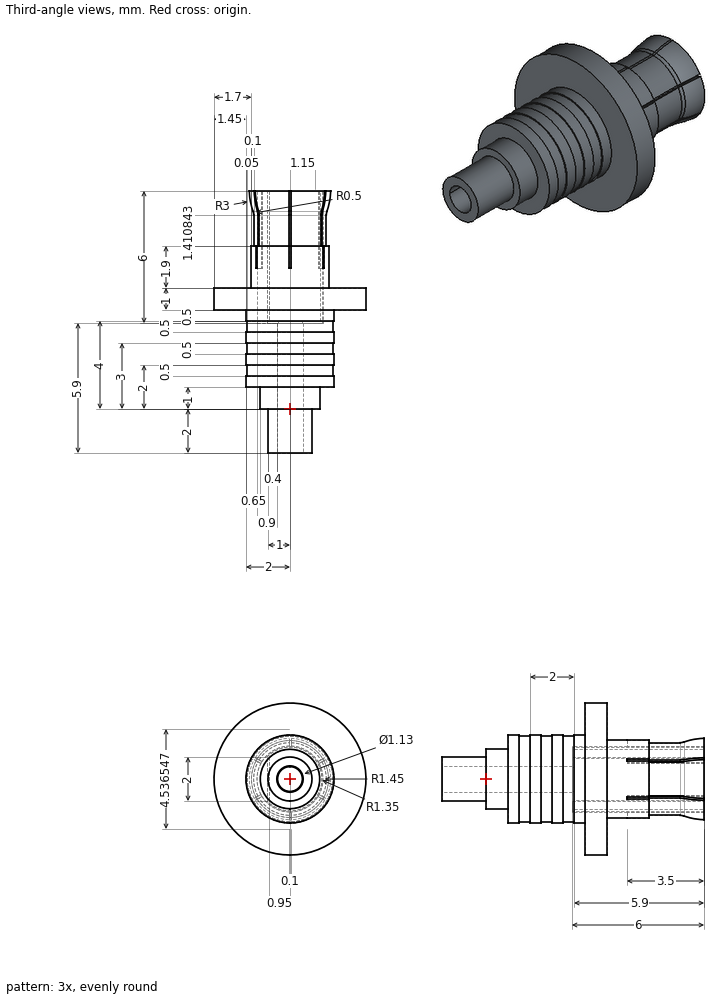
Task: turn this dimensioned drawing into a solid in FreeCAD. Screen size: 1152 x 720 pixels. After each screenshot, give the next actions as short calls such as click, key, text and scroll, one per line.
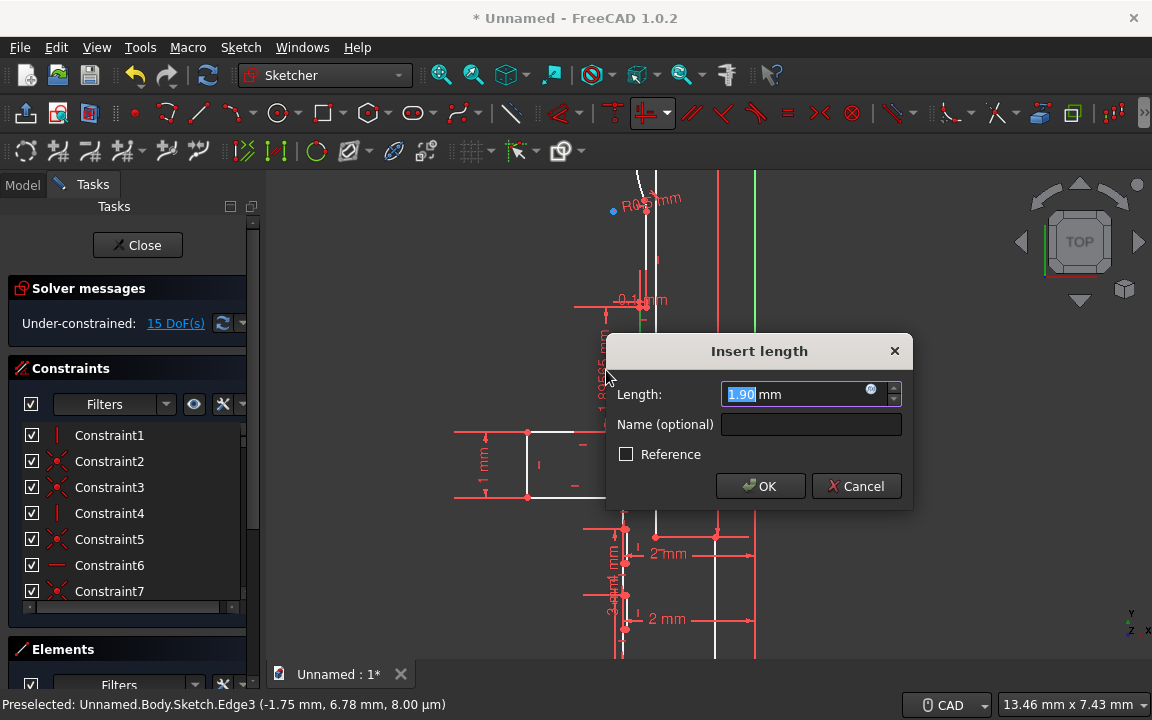
text(1.9)
key(Return)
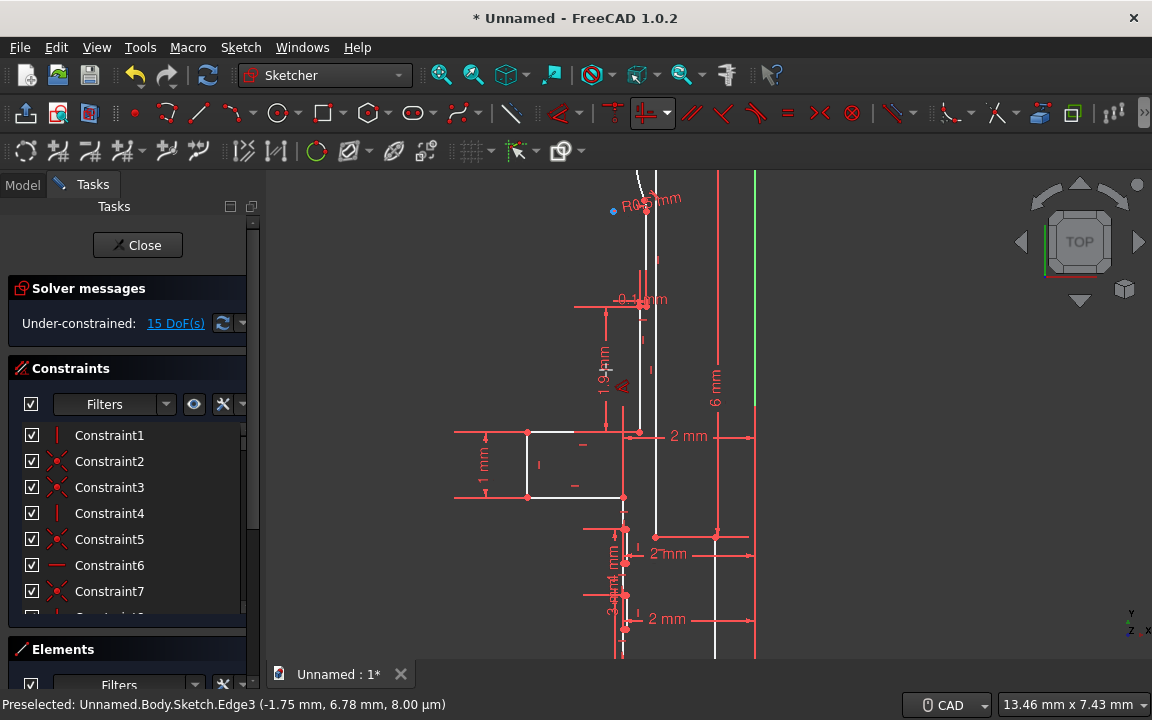
click(606, 432)
click(583, 398)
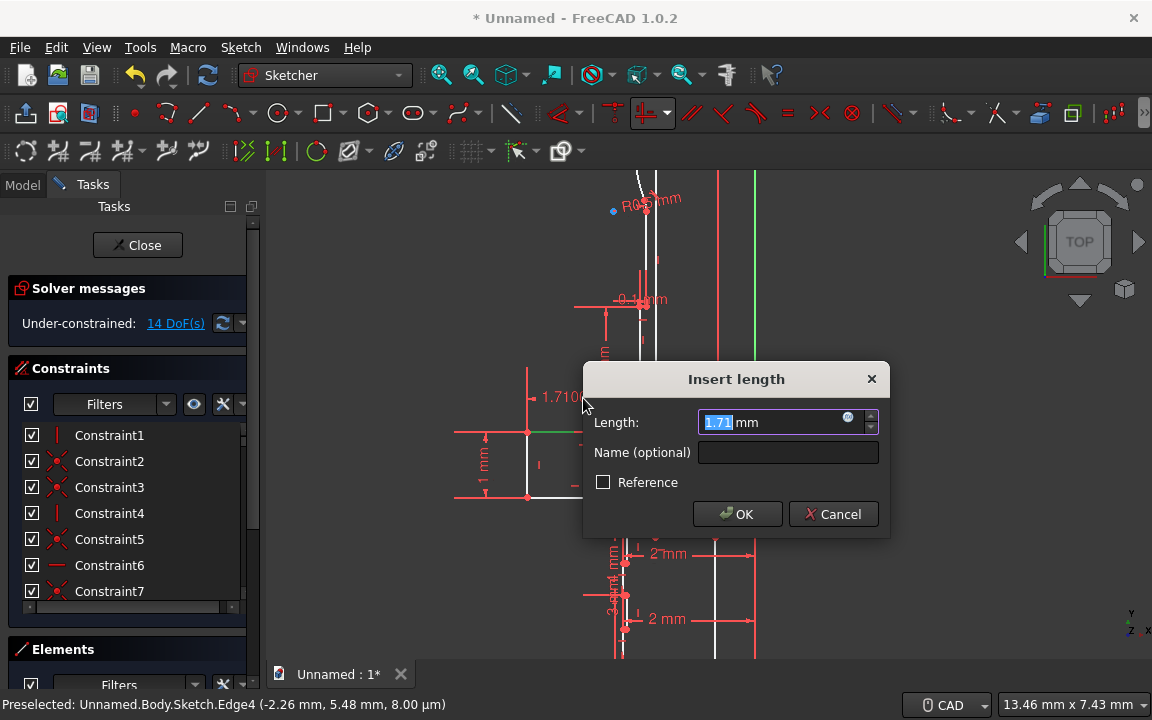
text(1.7)
key(Return)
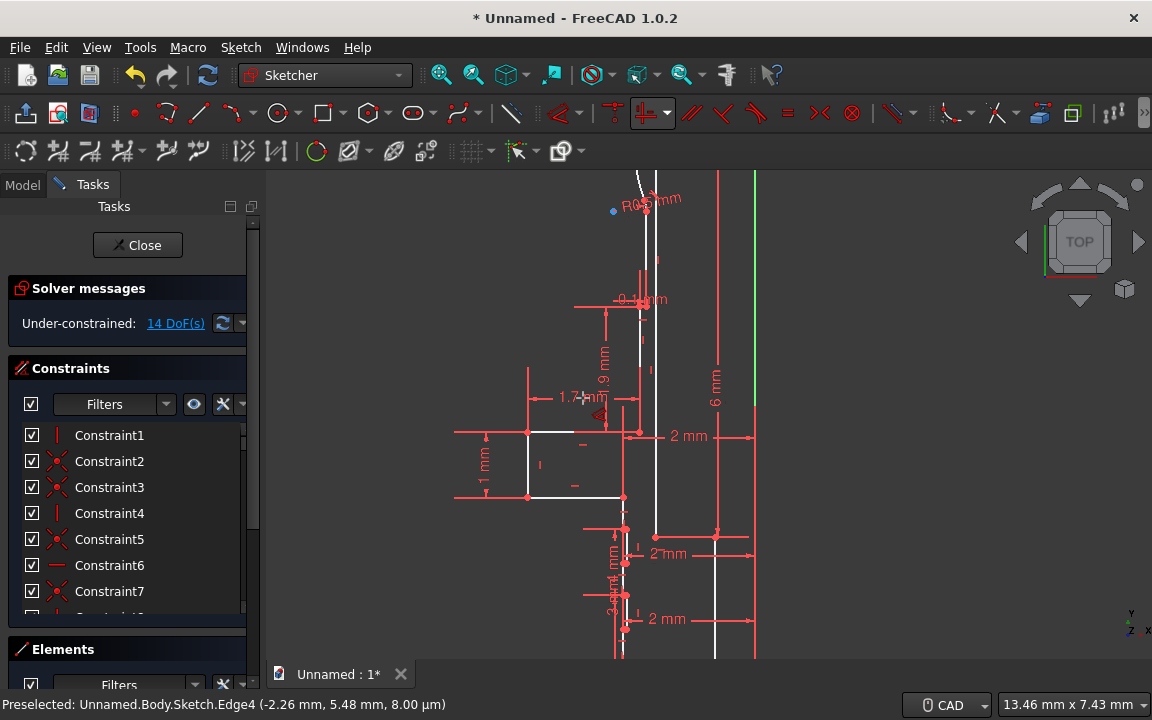
scroll(623, 507, up, 2)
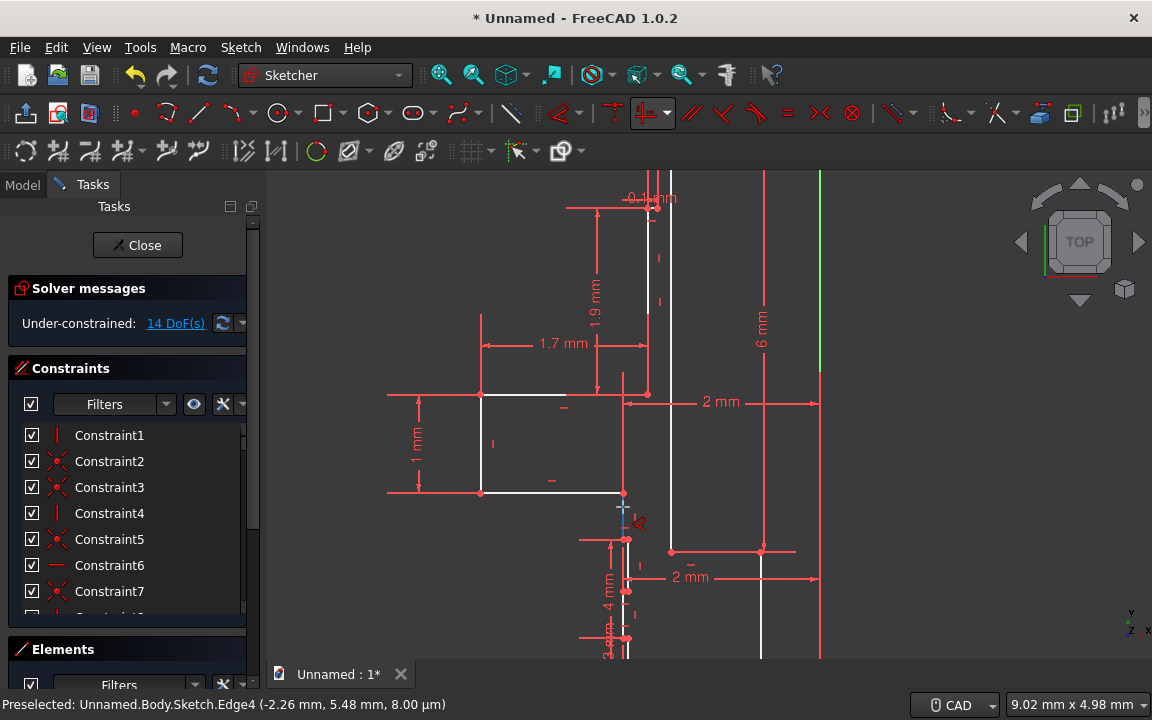
click(623, 507)
click(589, 516)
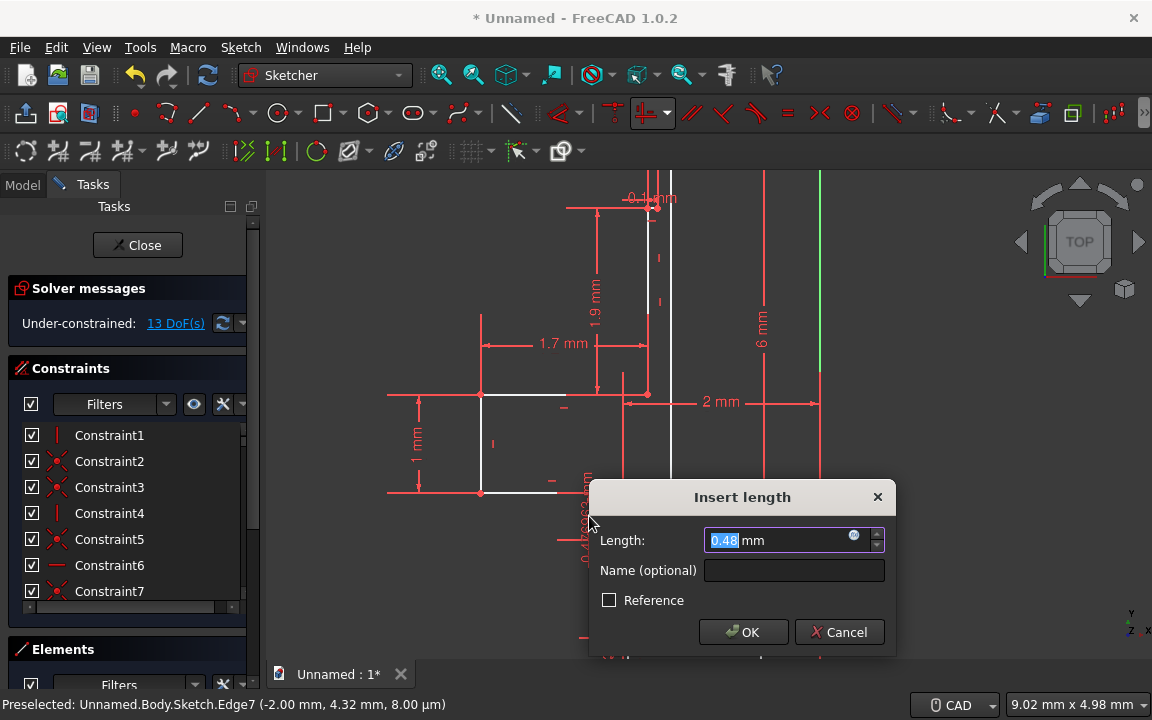
text(0.5)
key(Return)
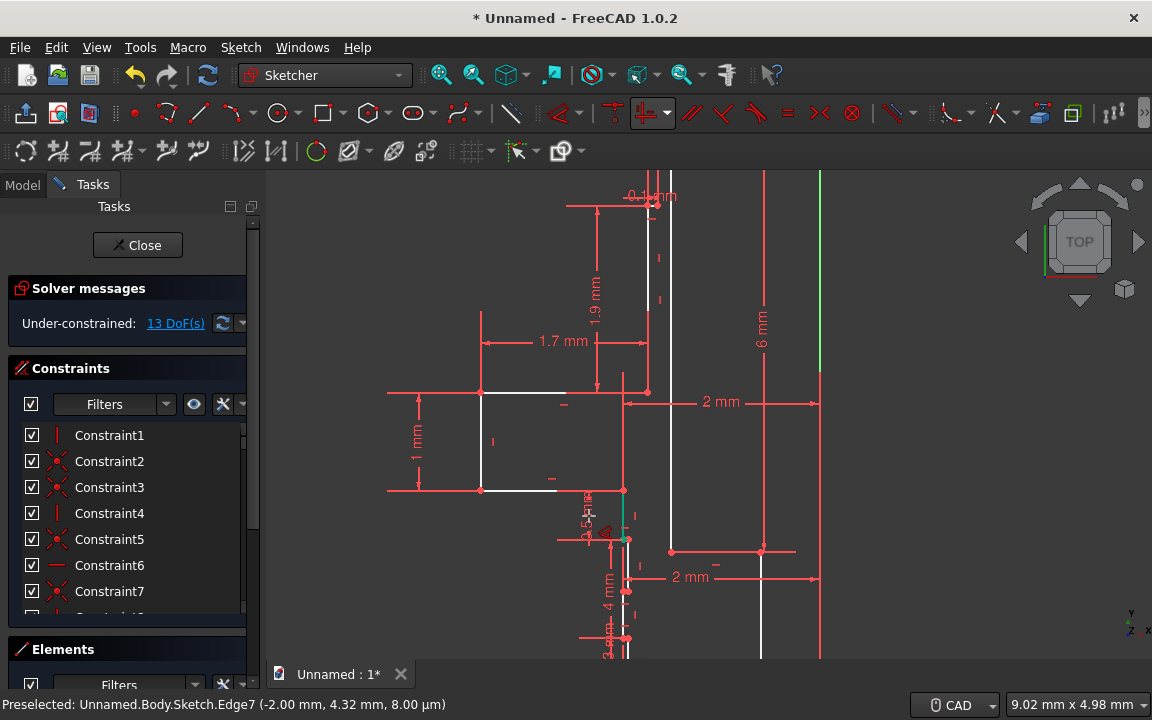
click(628, 555)
click(594, 566)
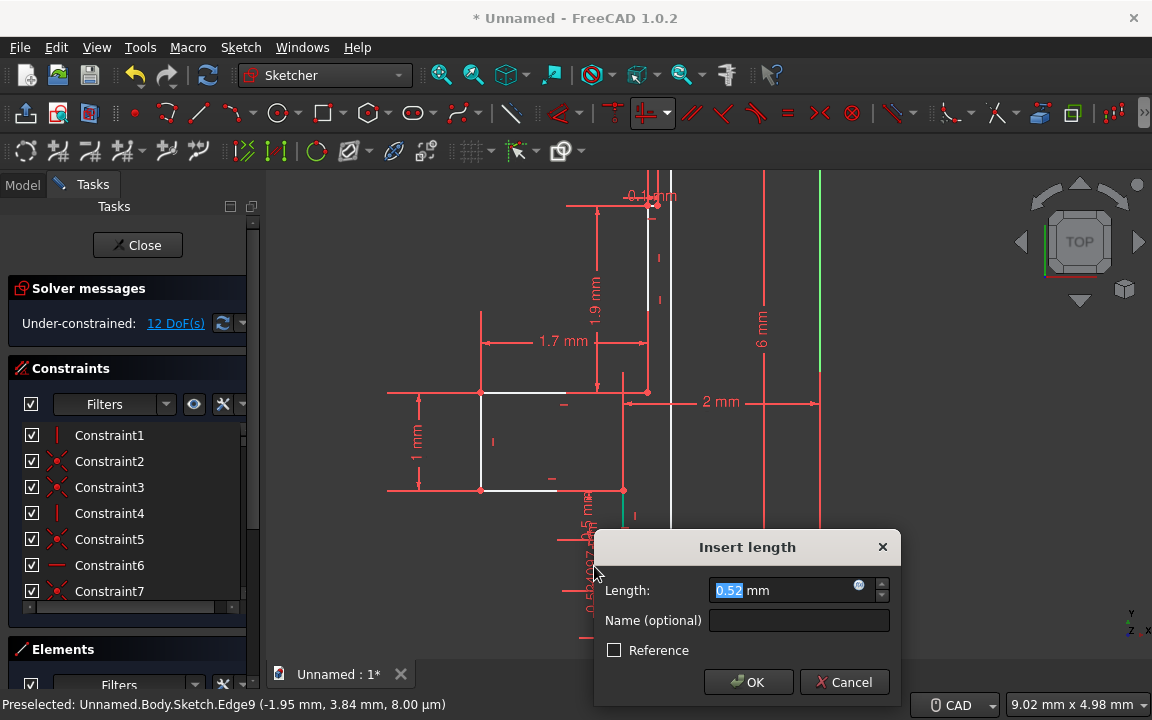
text(0.5)
key(Return)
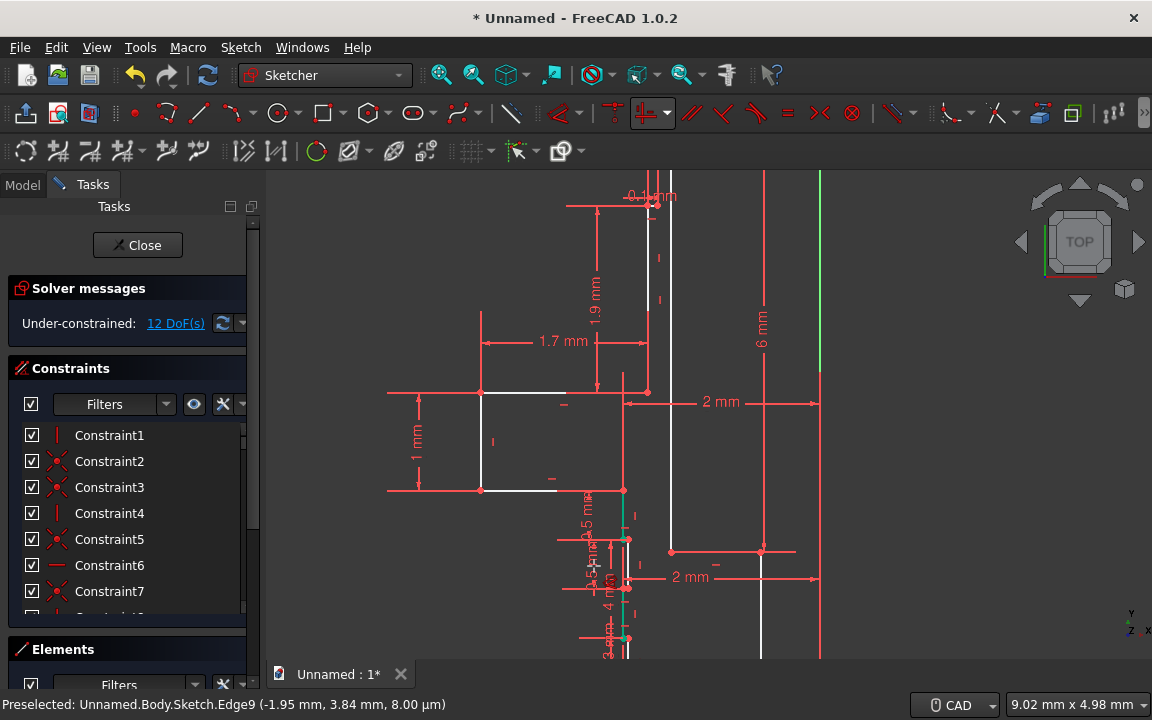
scroll(637, 372, down, 7)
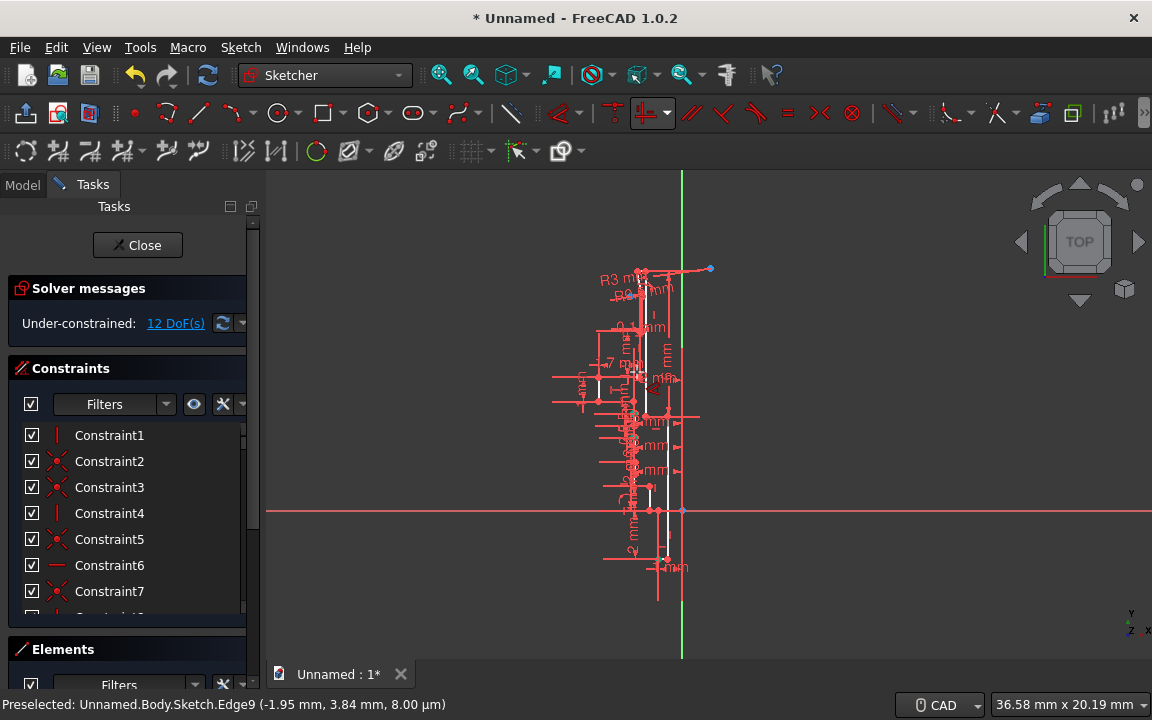
scroll(635, 442, up, 7)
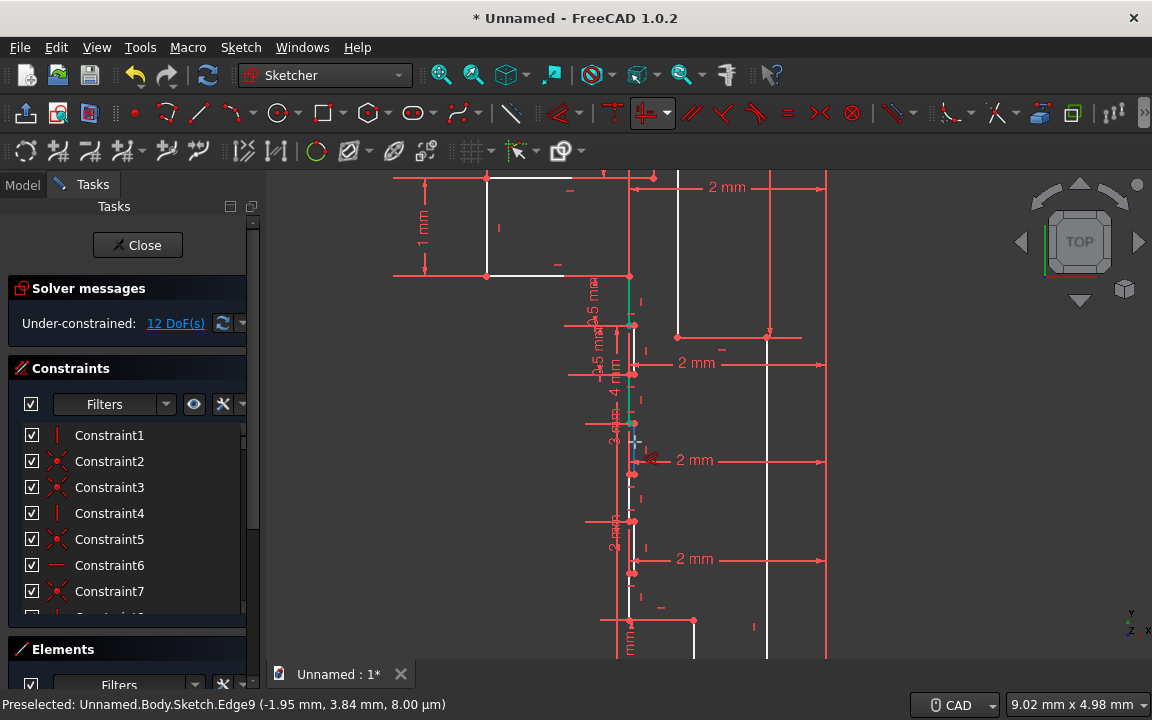
click(634, 439)
click(600, 449)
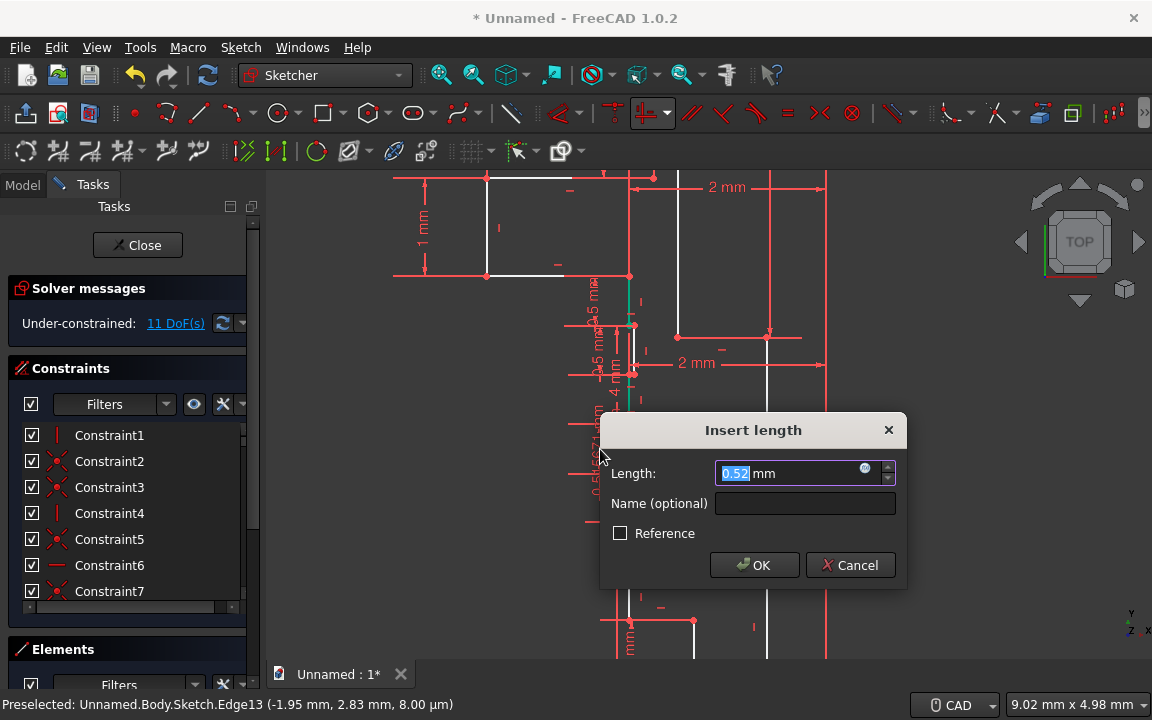
text(0.5)
key(Return)